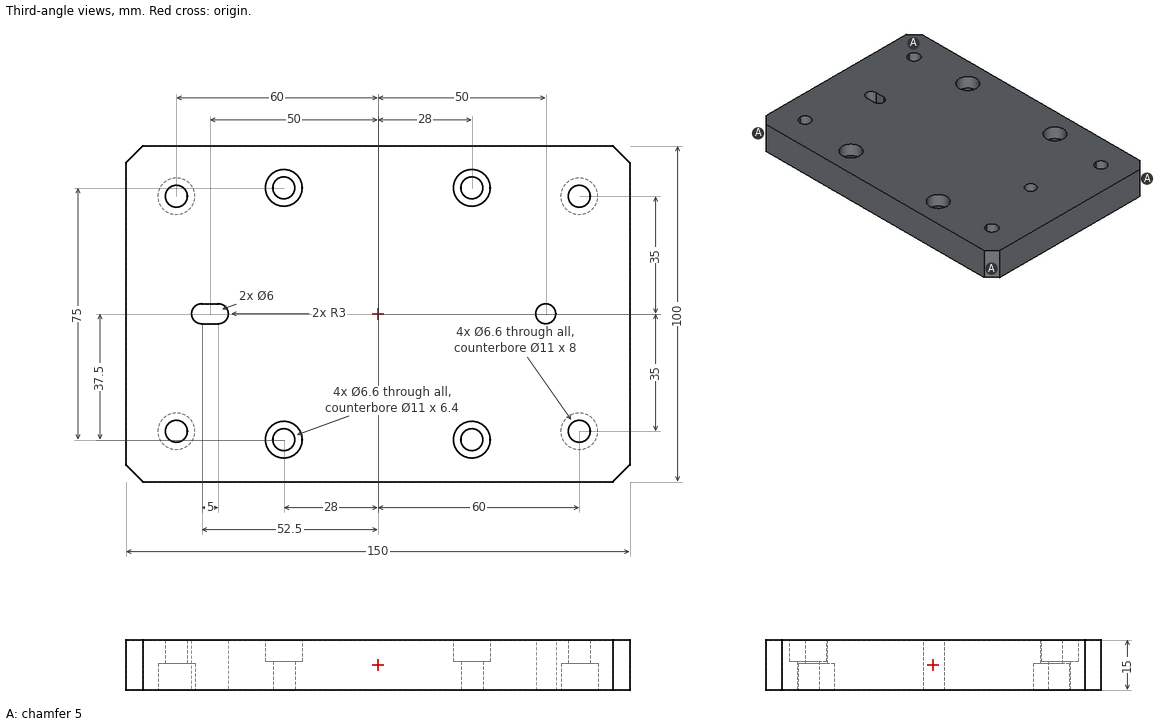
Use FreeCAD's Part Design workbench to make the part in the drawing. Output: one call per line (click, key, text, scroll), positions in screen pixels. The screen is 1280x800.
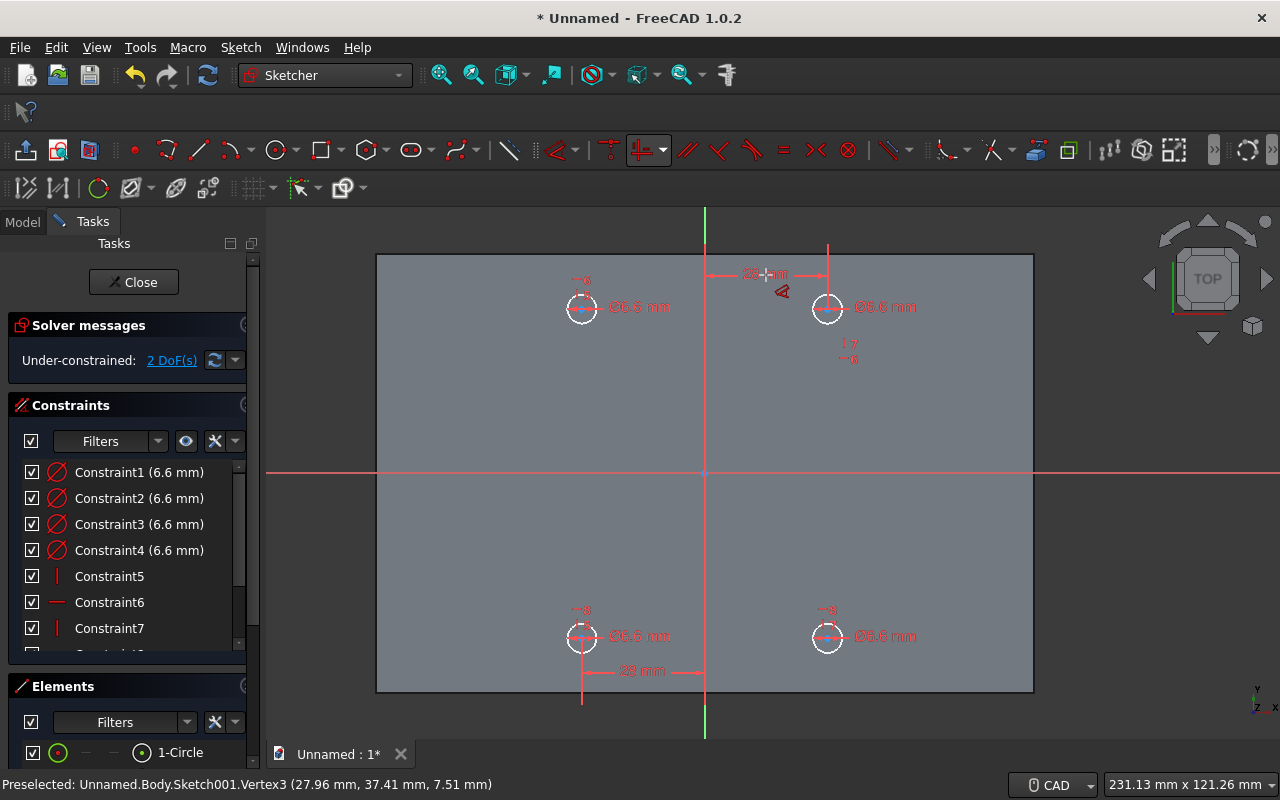
click(582, 638)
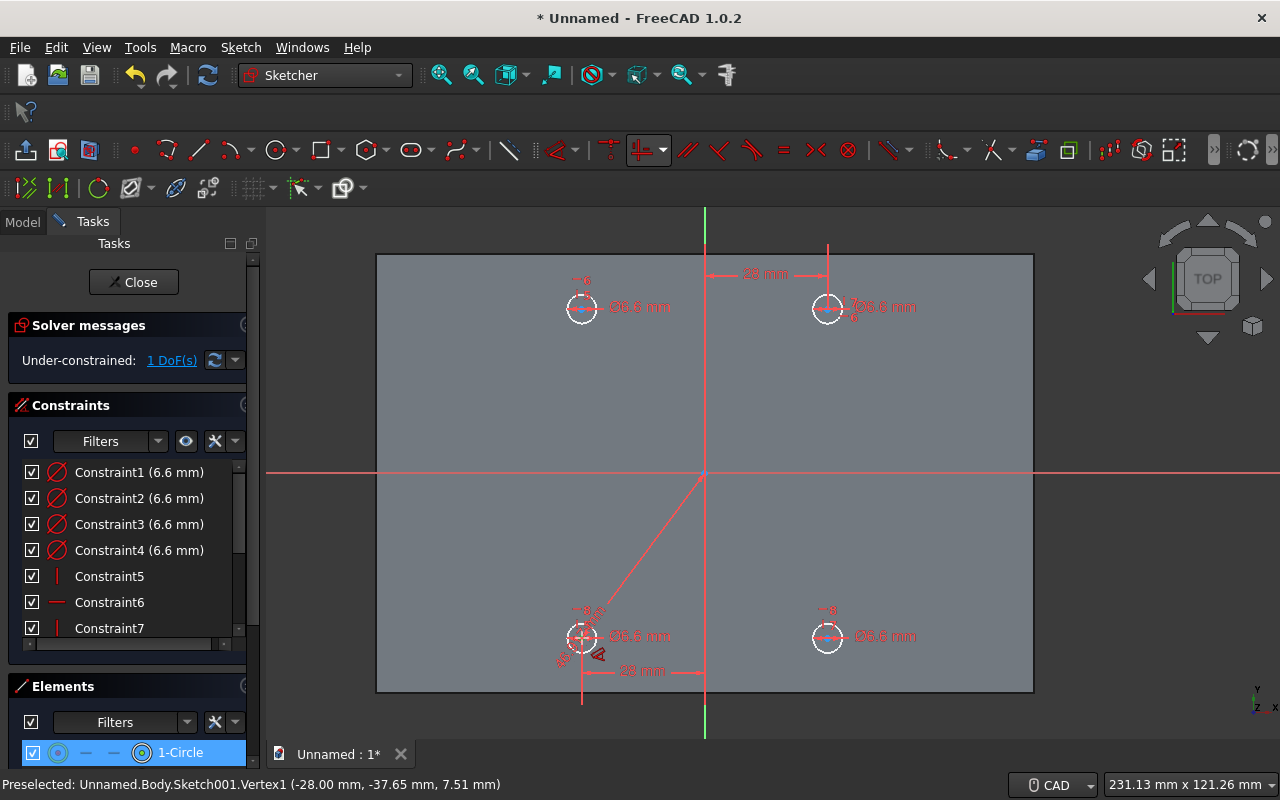
click(582, 309)
click(548, 398)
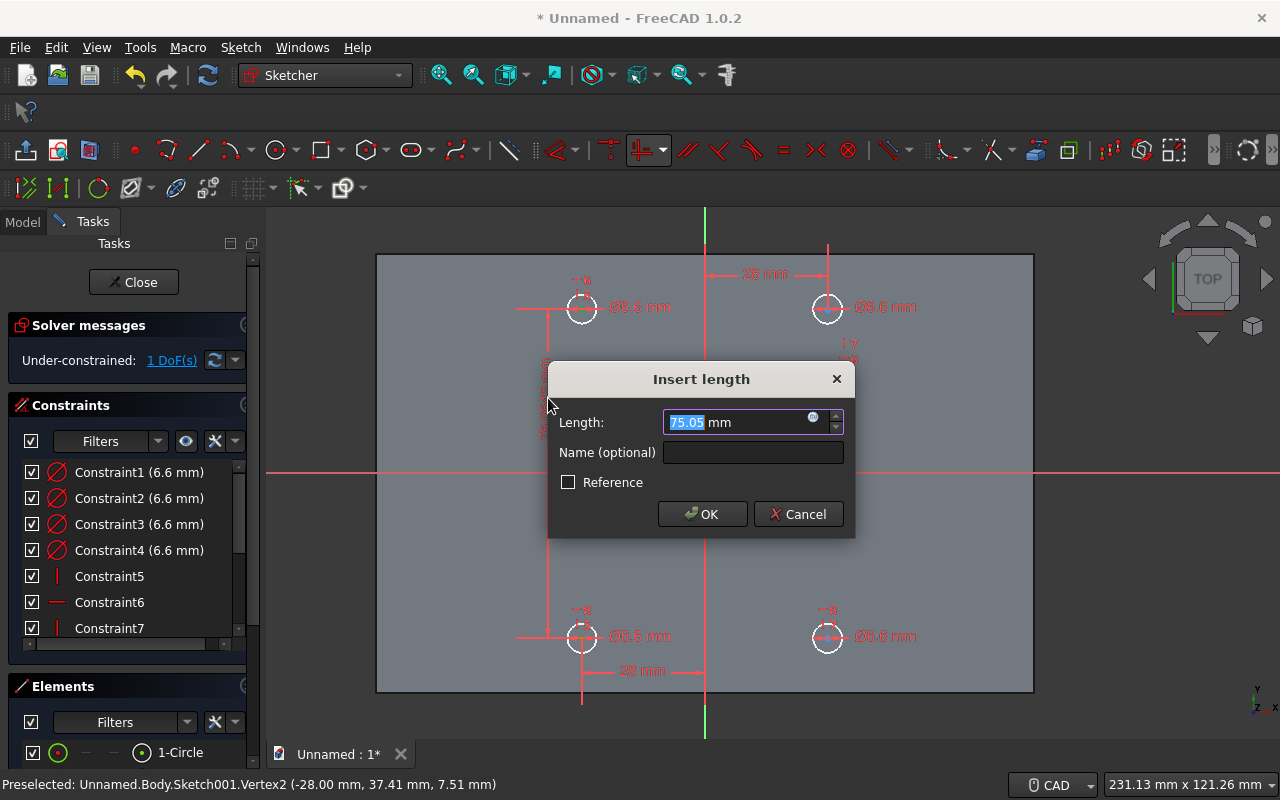
text(75)
key(Return)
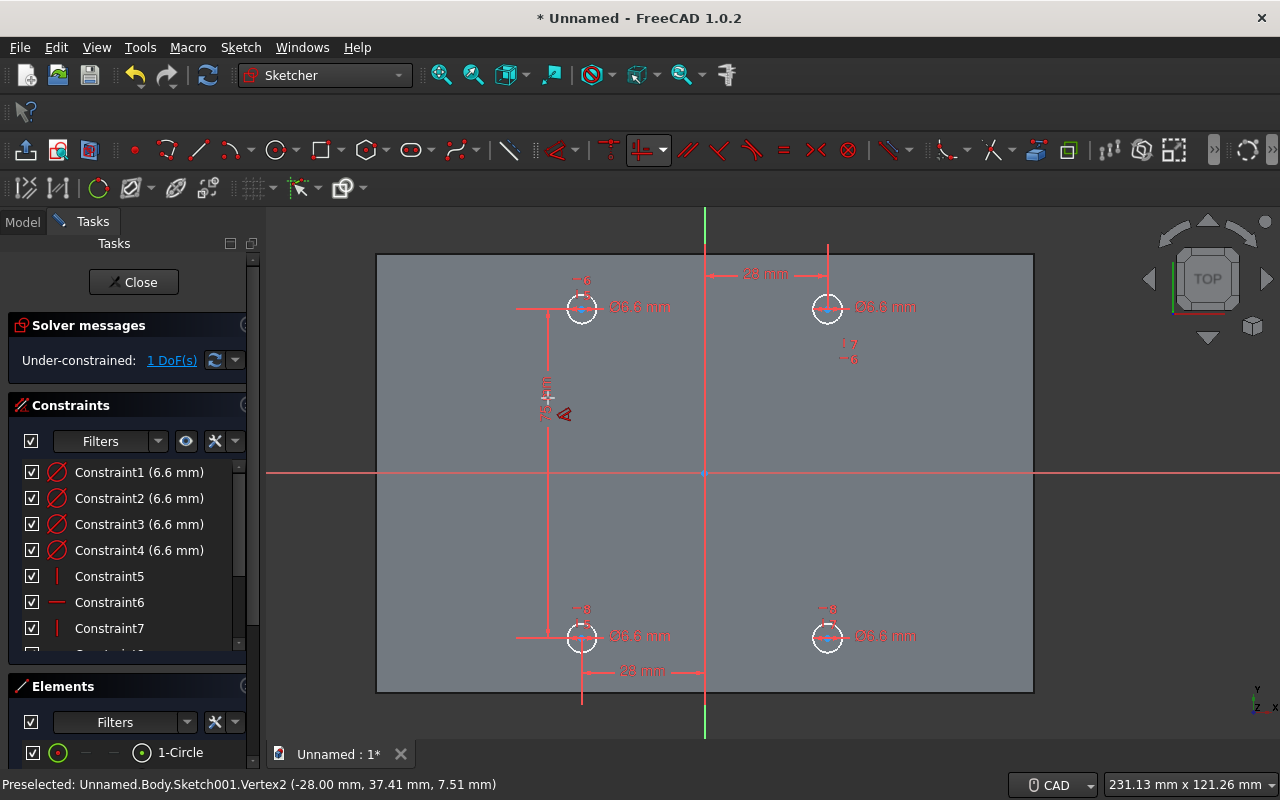
click(582, 638)
click(548, 556)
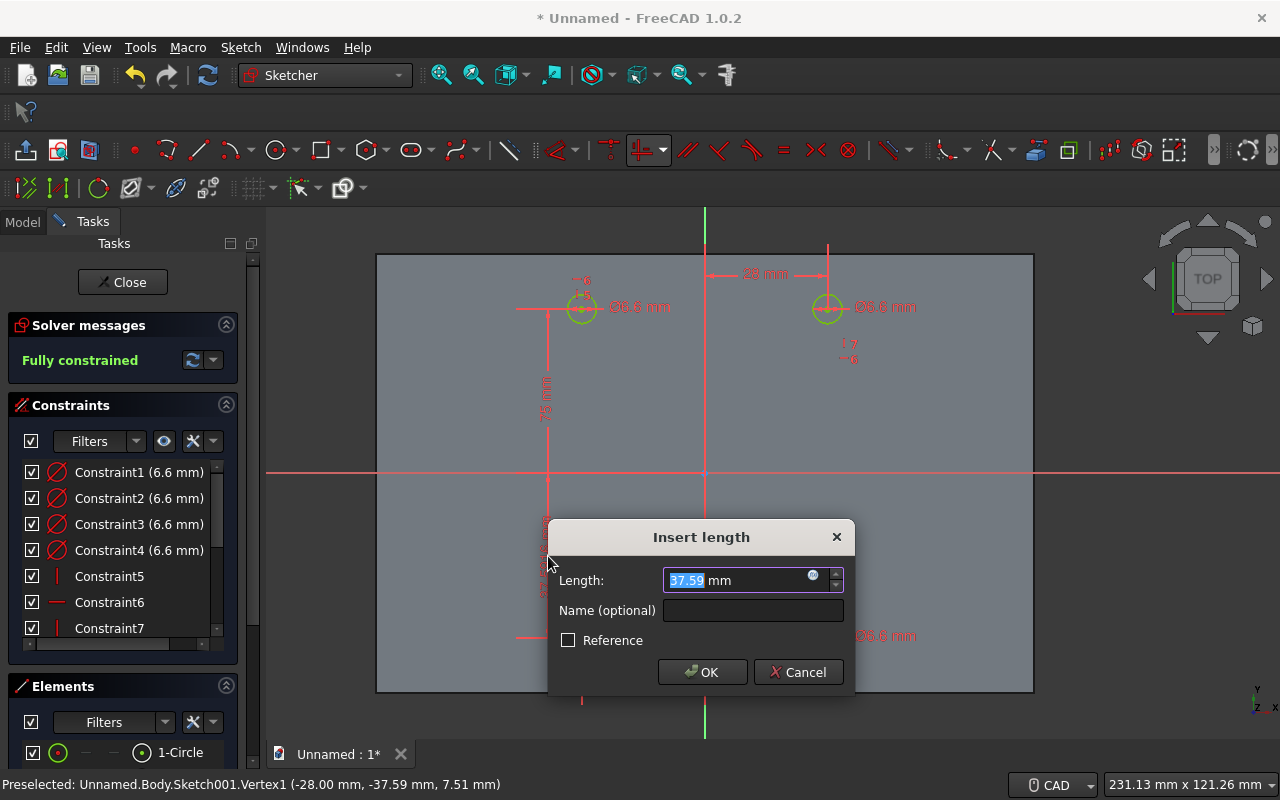
text(37.5)
key(Return)
key(Escape)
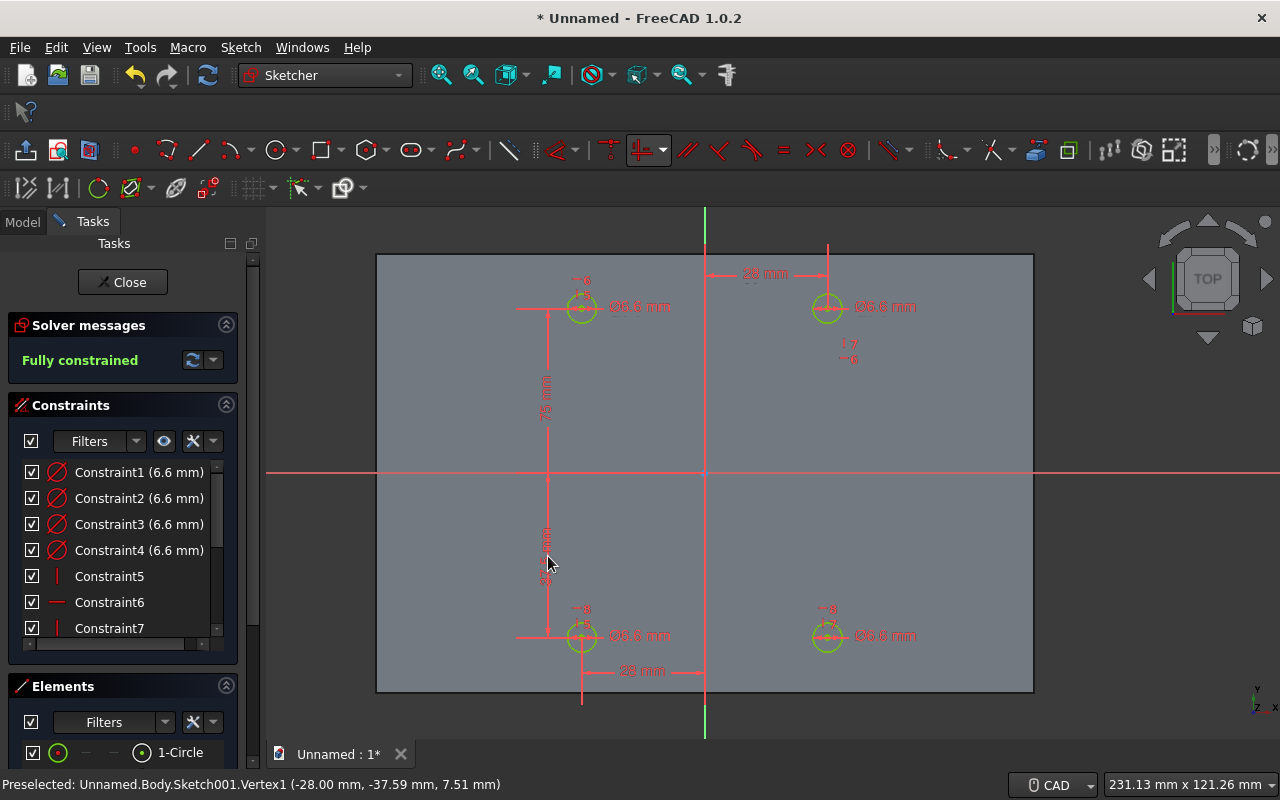
click(123, 282)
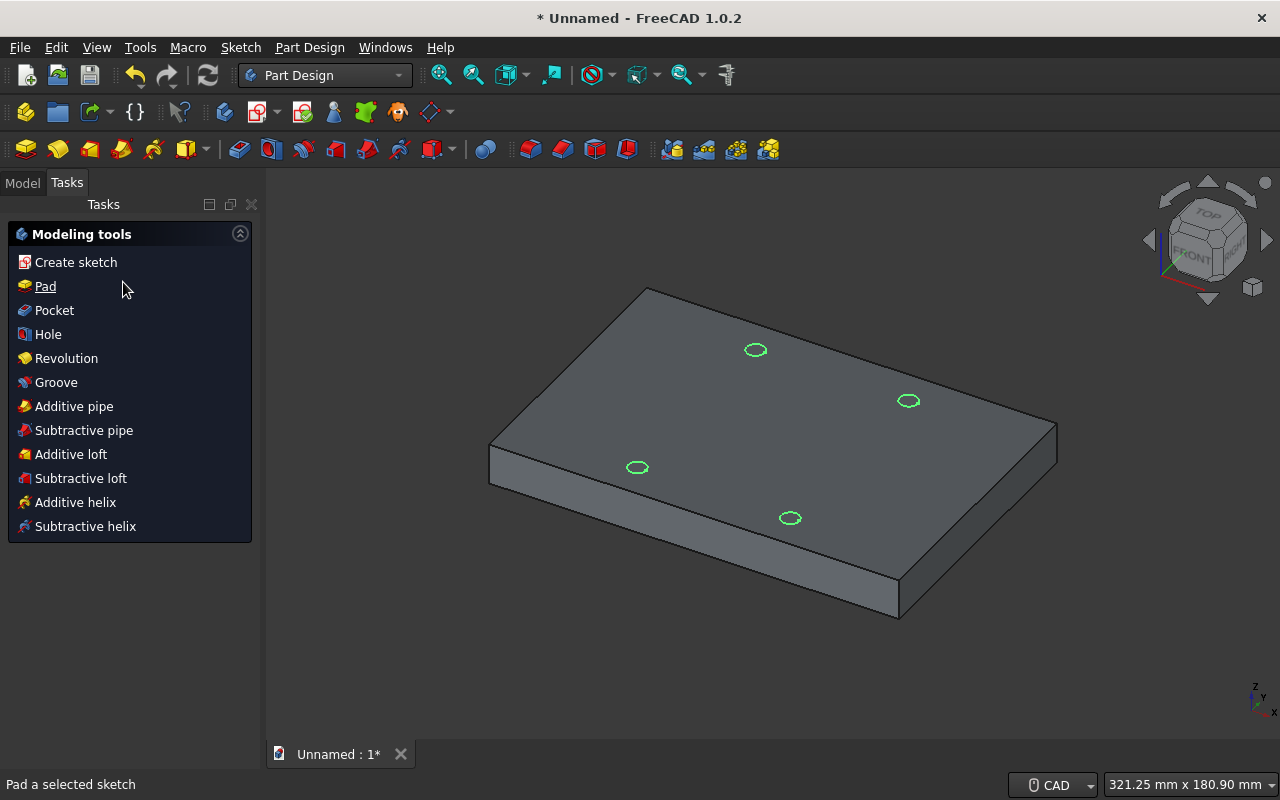
click(272, 150)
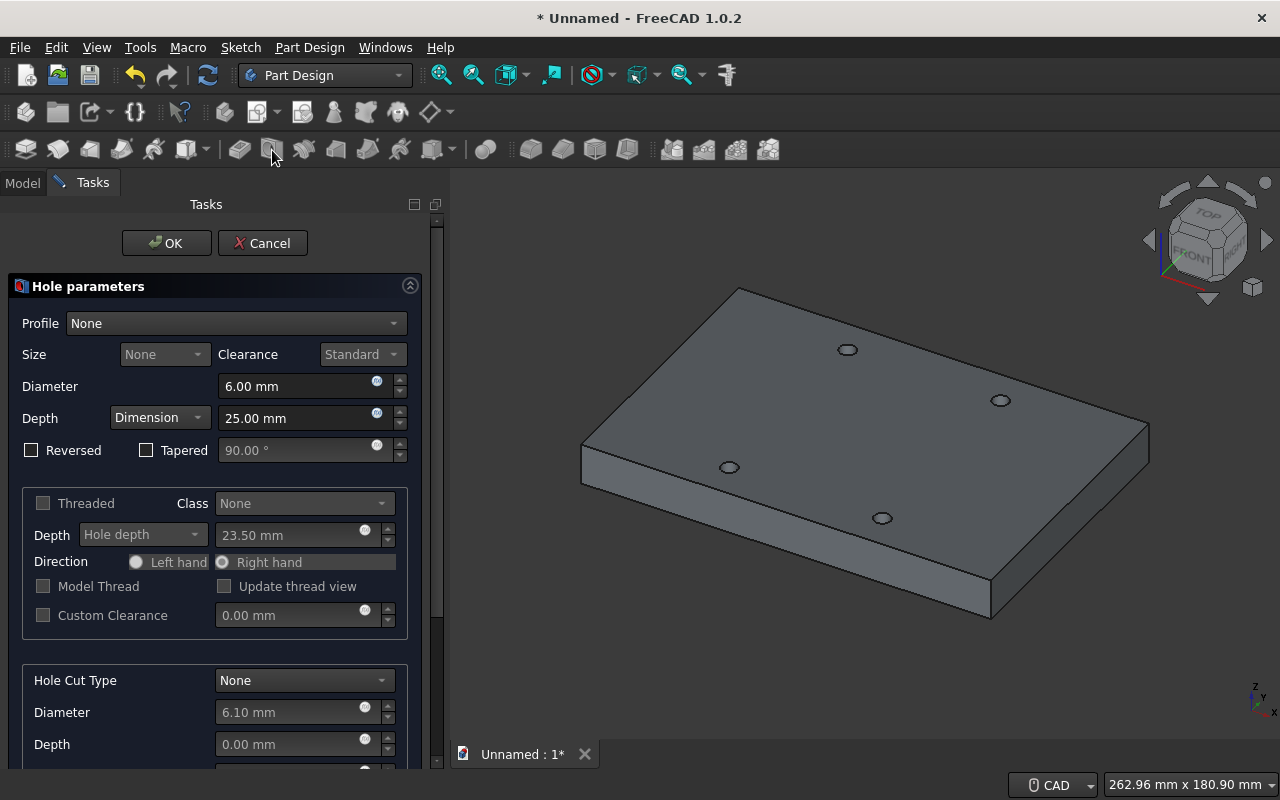
triple_click(305, 386)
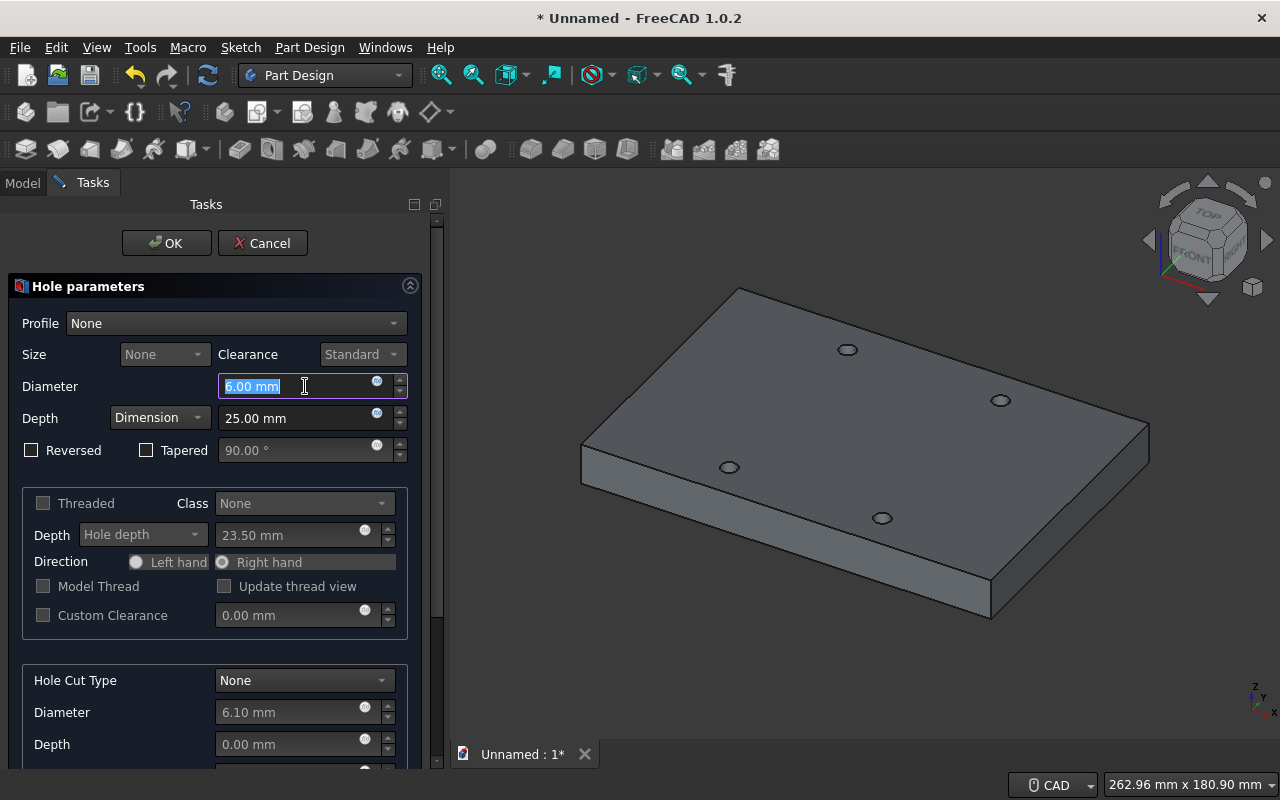
text(6.6)
key(Tab)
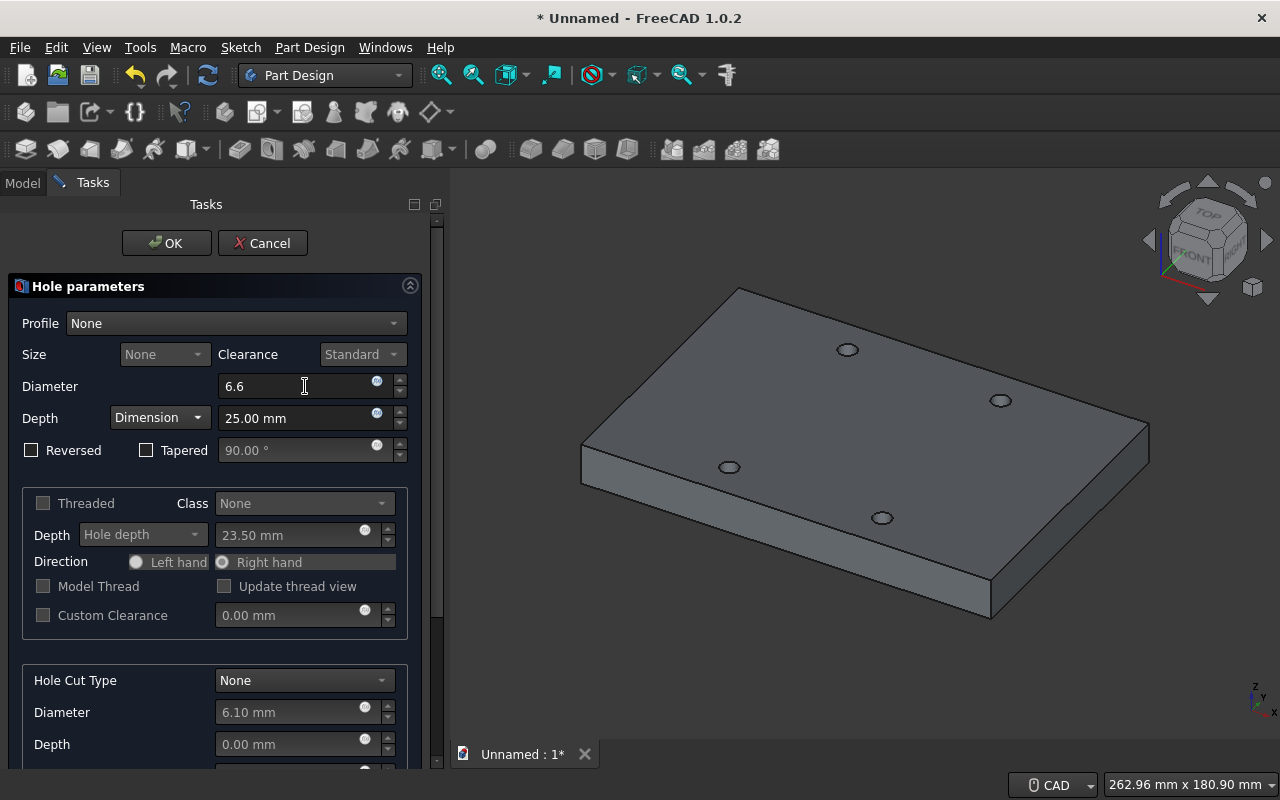
click(161, 418)